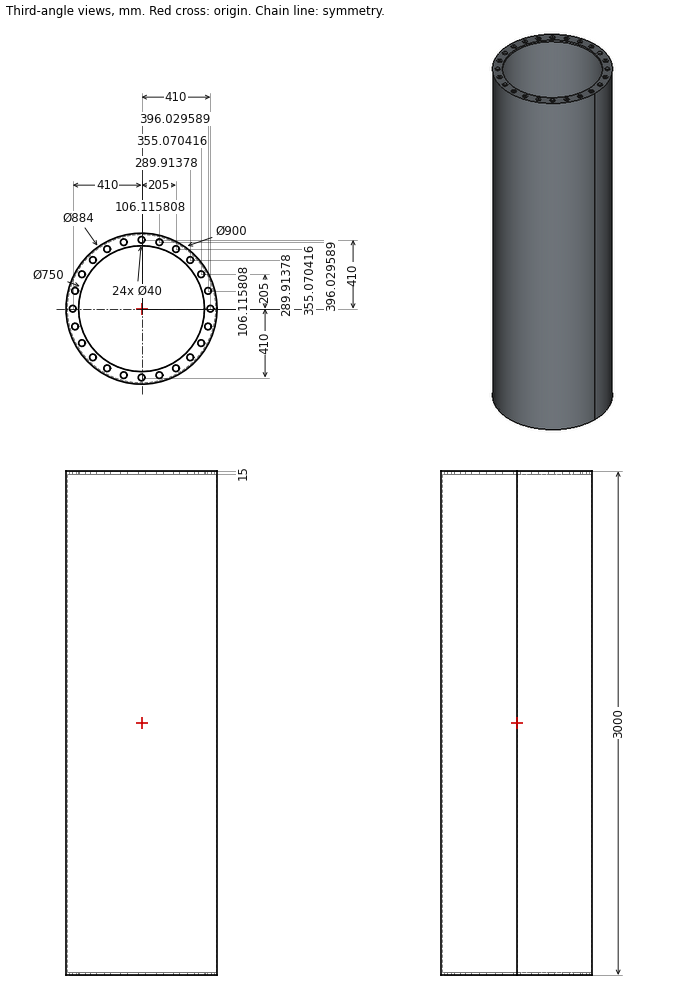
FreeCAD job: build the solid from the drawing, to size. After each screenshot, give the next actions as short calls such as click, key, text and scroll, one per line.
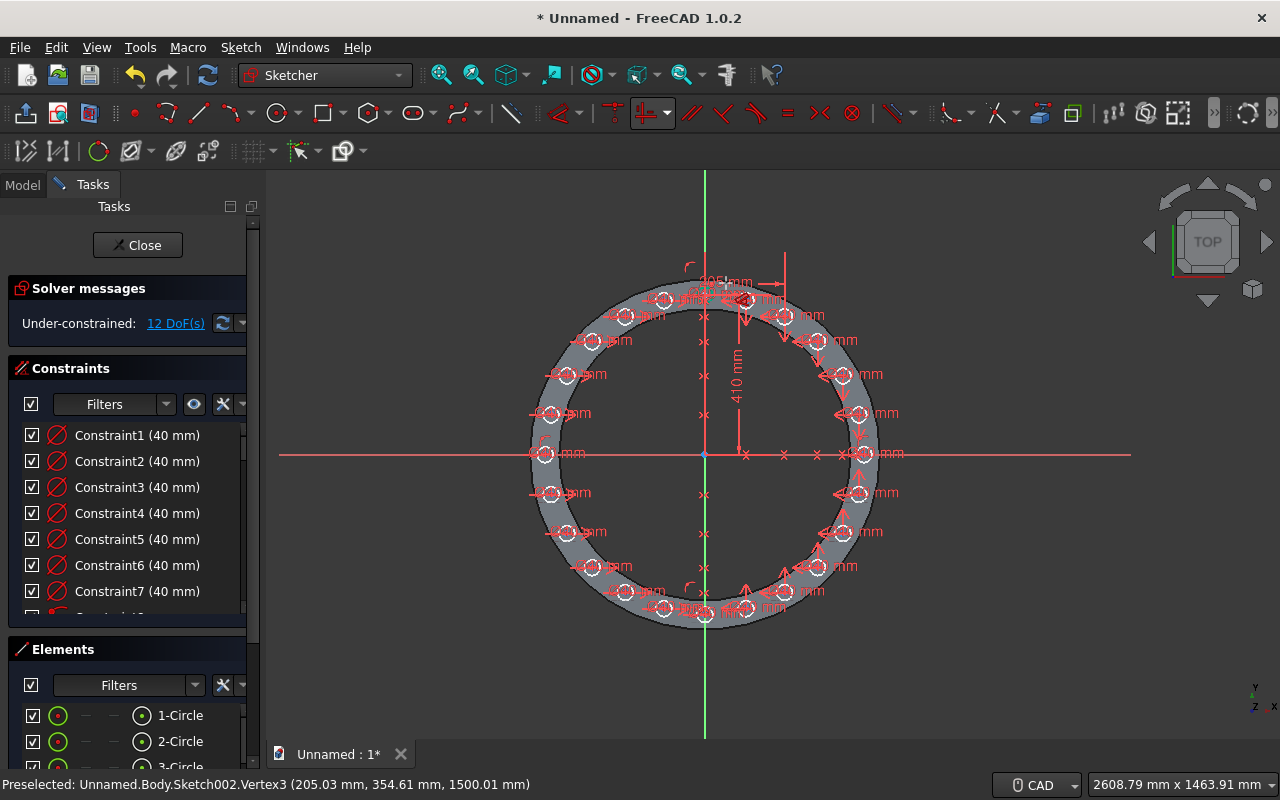
click(843, 376)
click(877, 397)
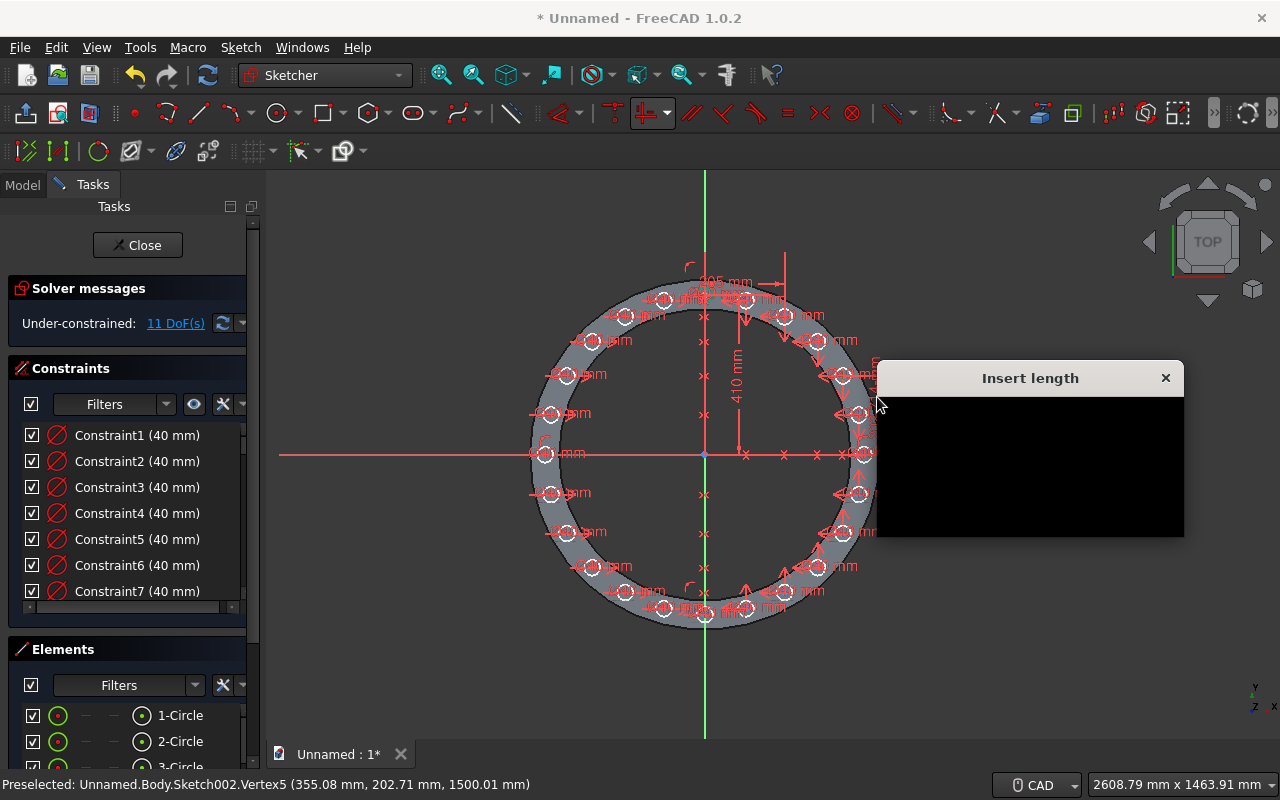
text(205)
key(Return)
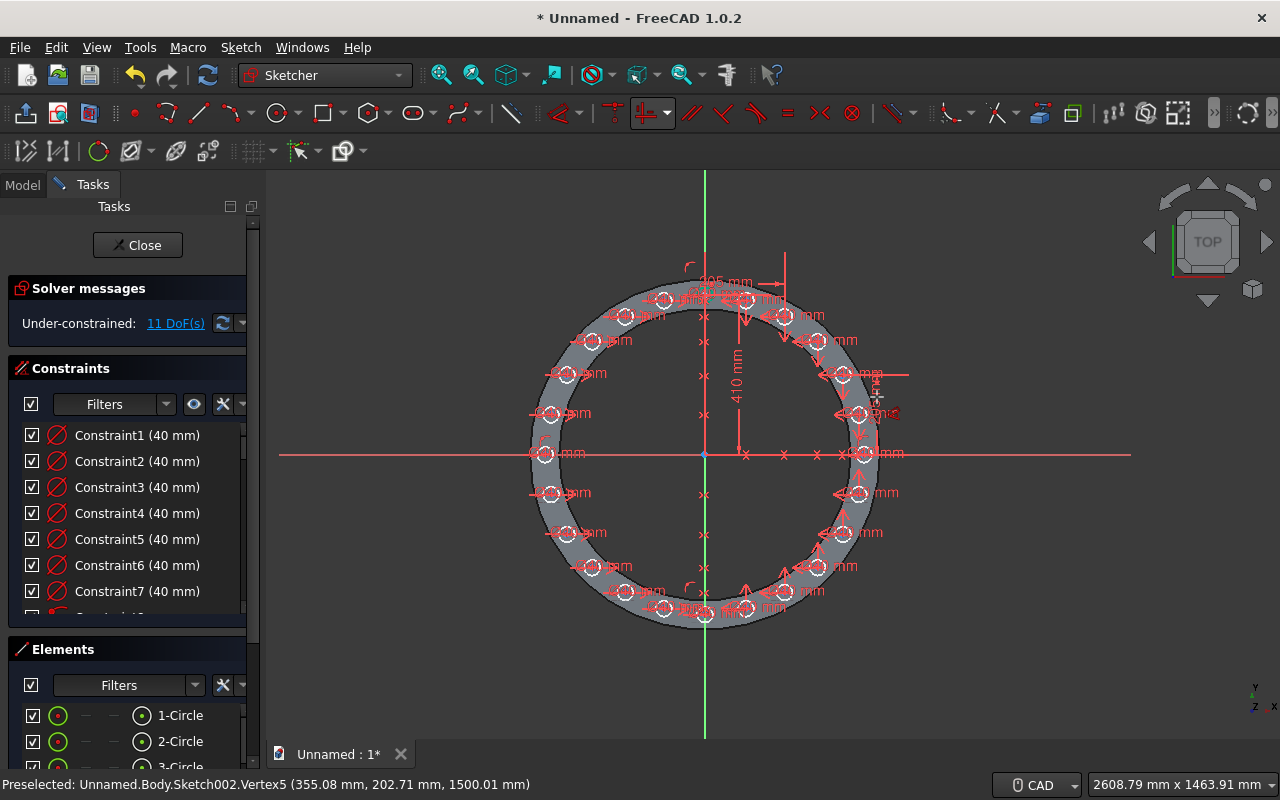
click(864, 455)
click(784, 489)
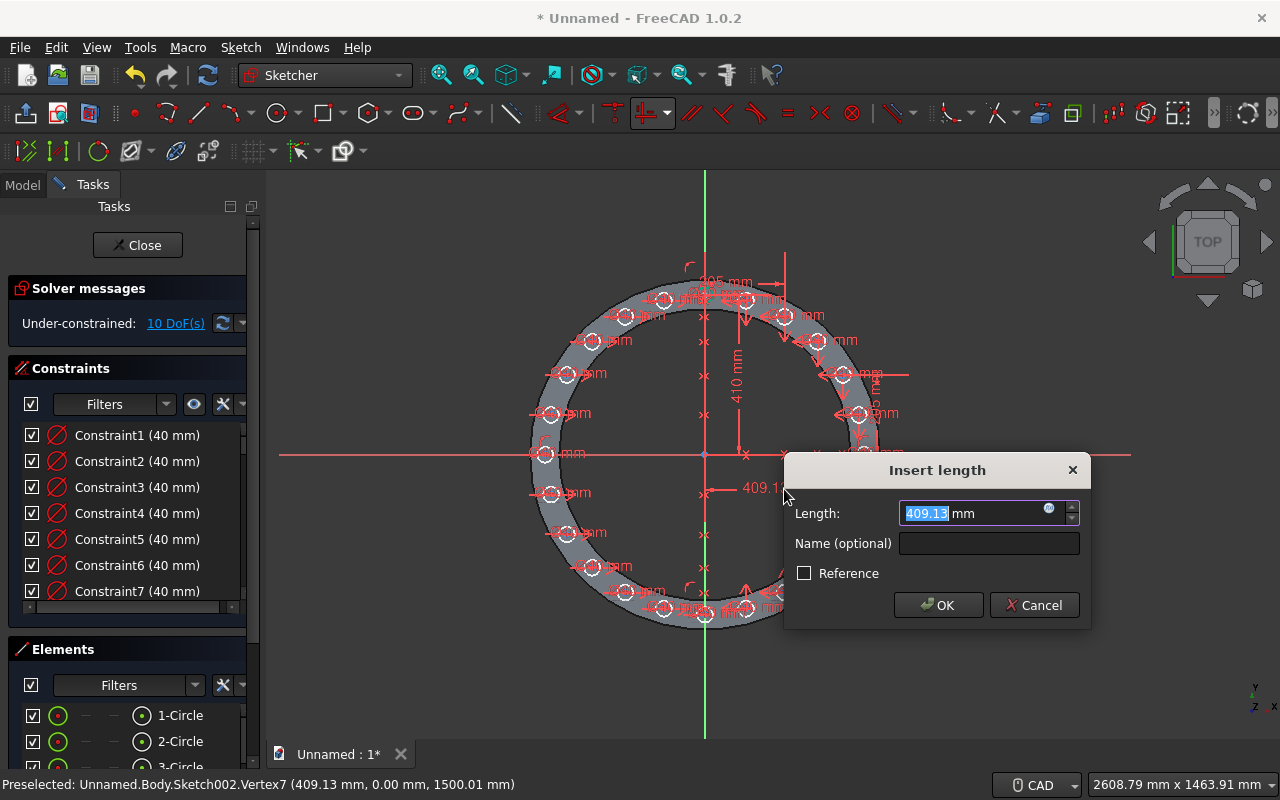
text(410)
key(Return)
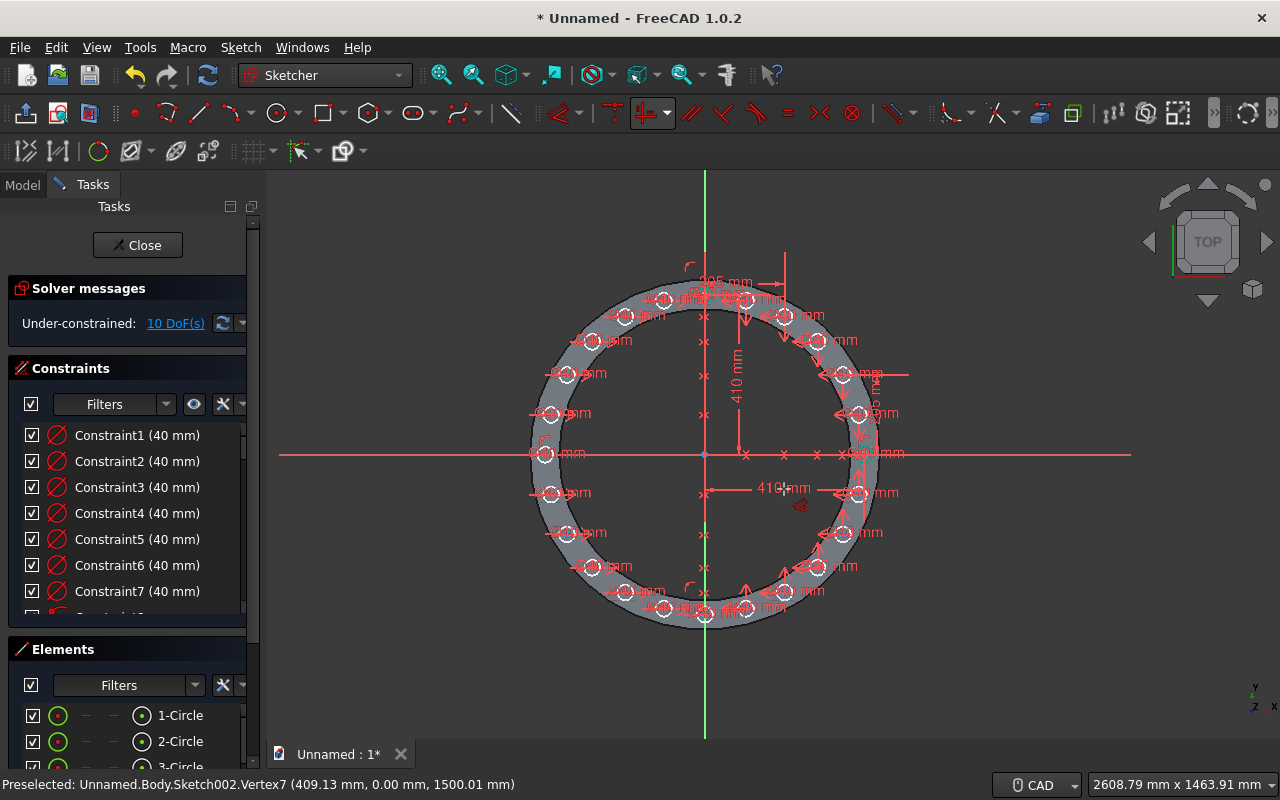
click(705, 615)
click(739, 535)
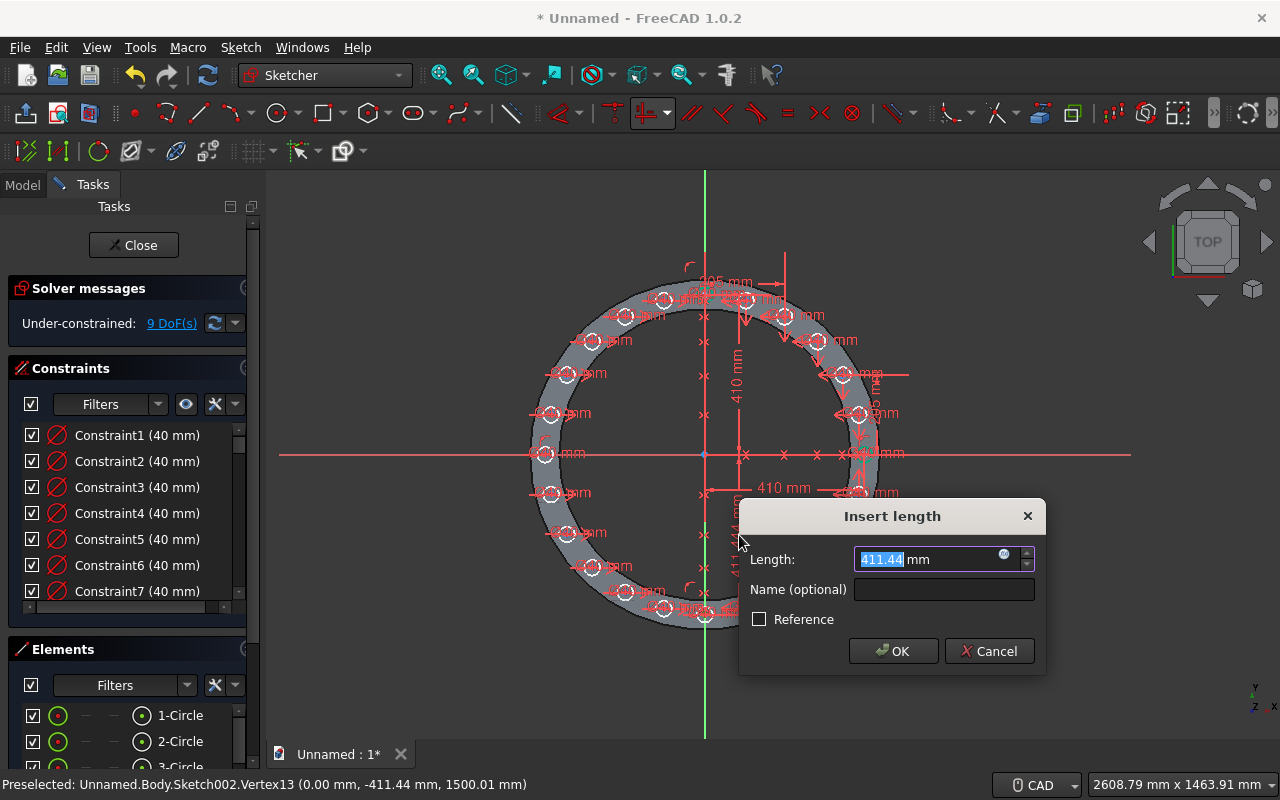
text(410)
key(Return)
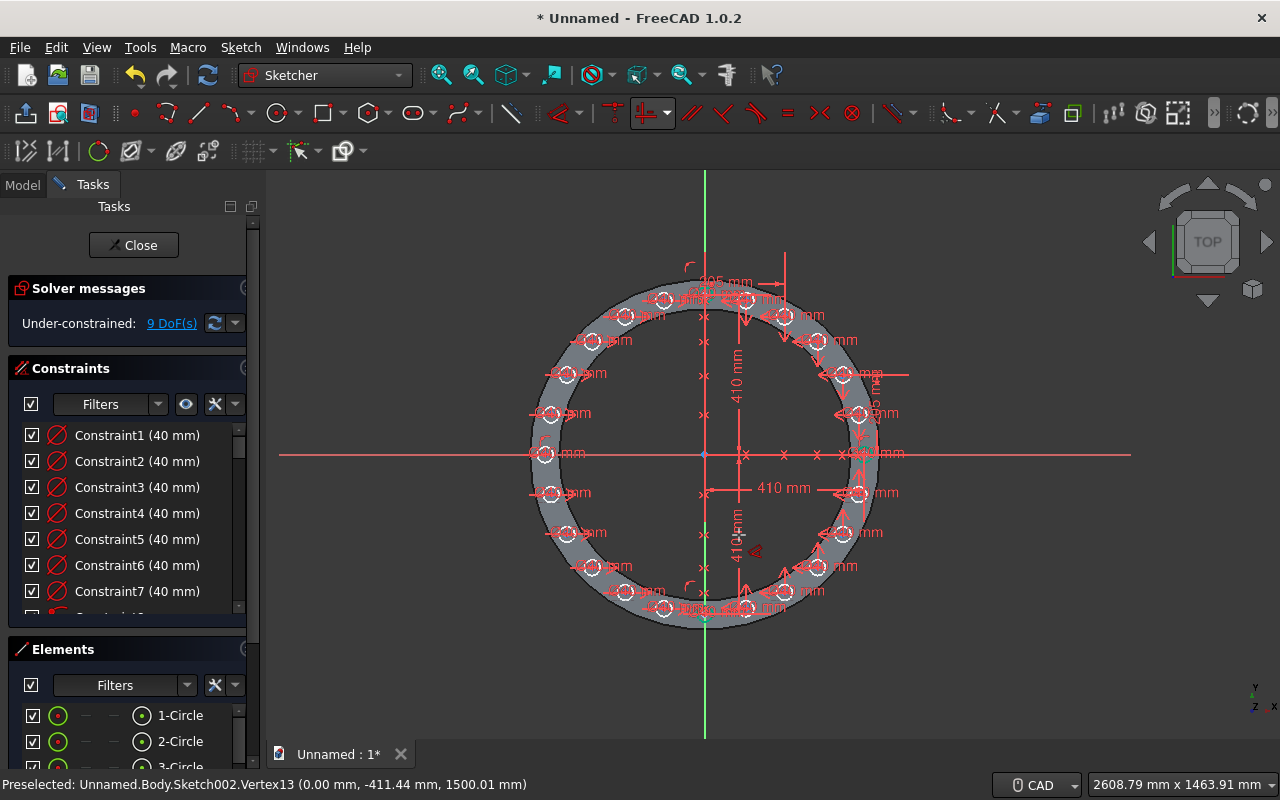
click(545, 455)
click(625, 489)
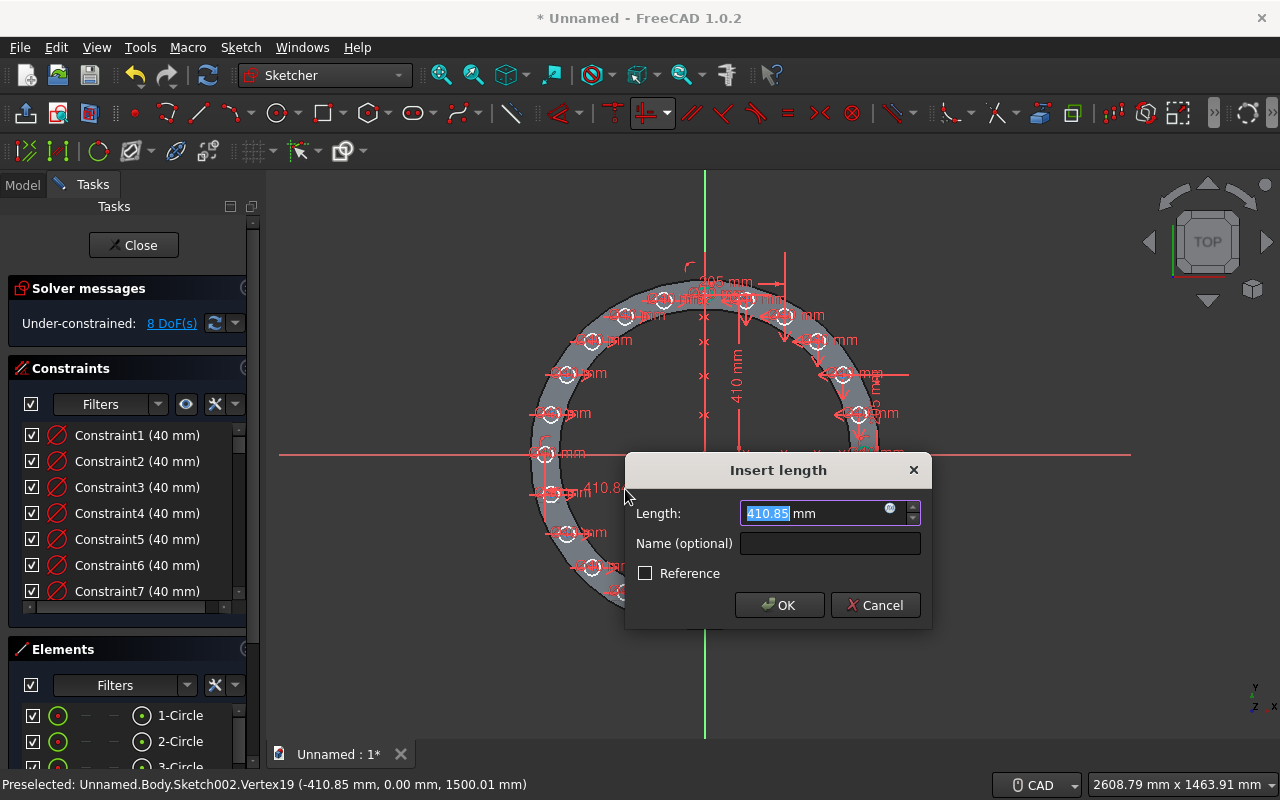
text(410)
key(Return)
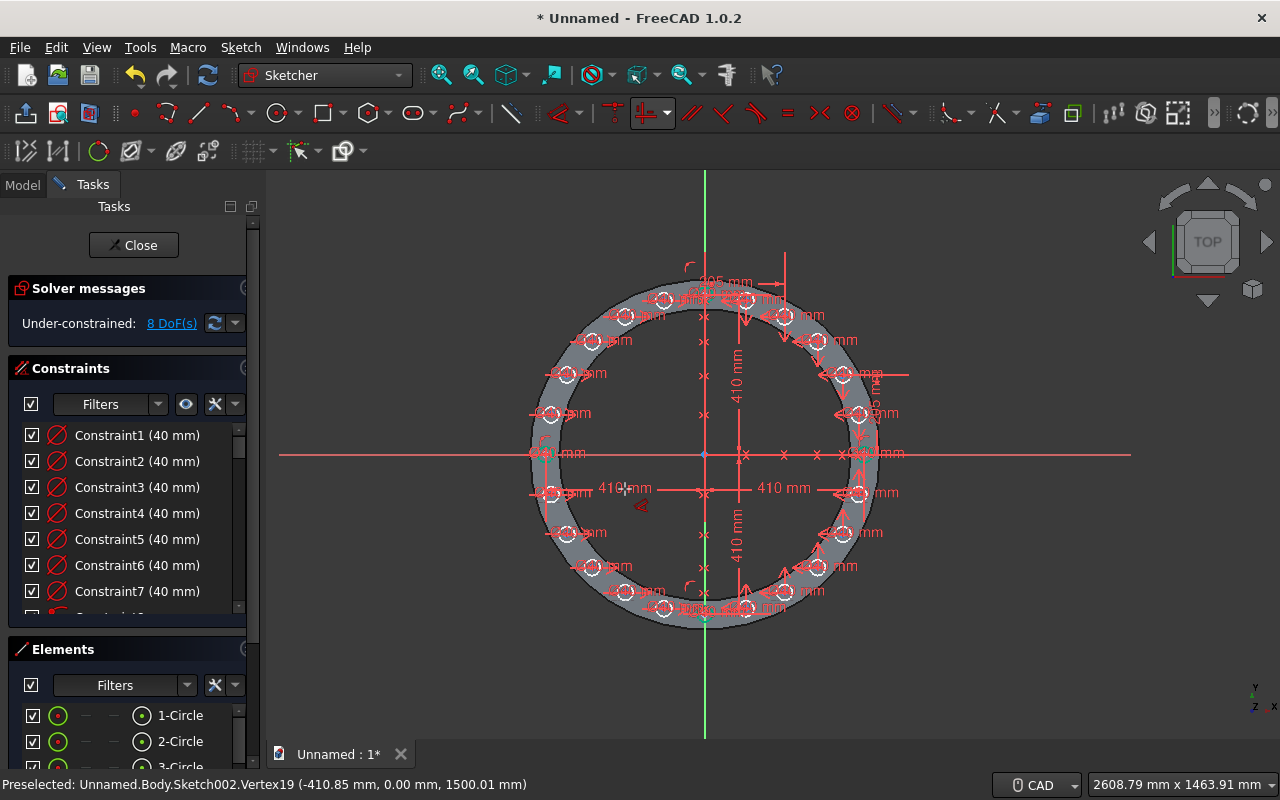
click(818, 342)
click(722, 308)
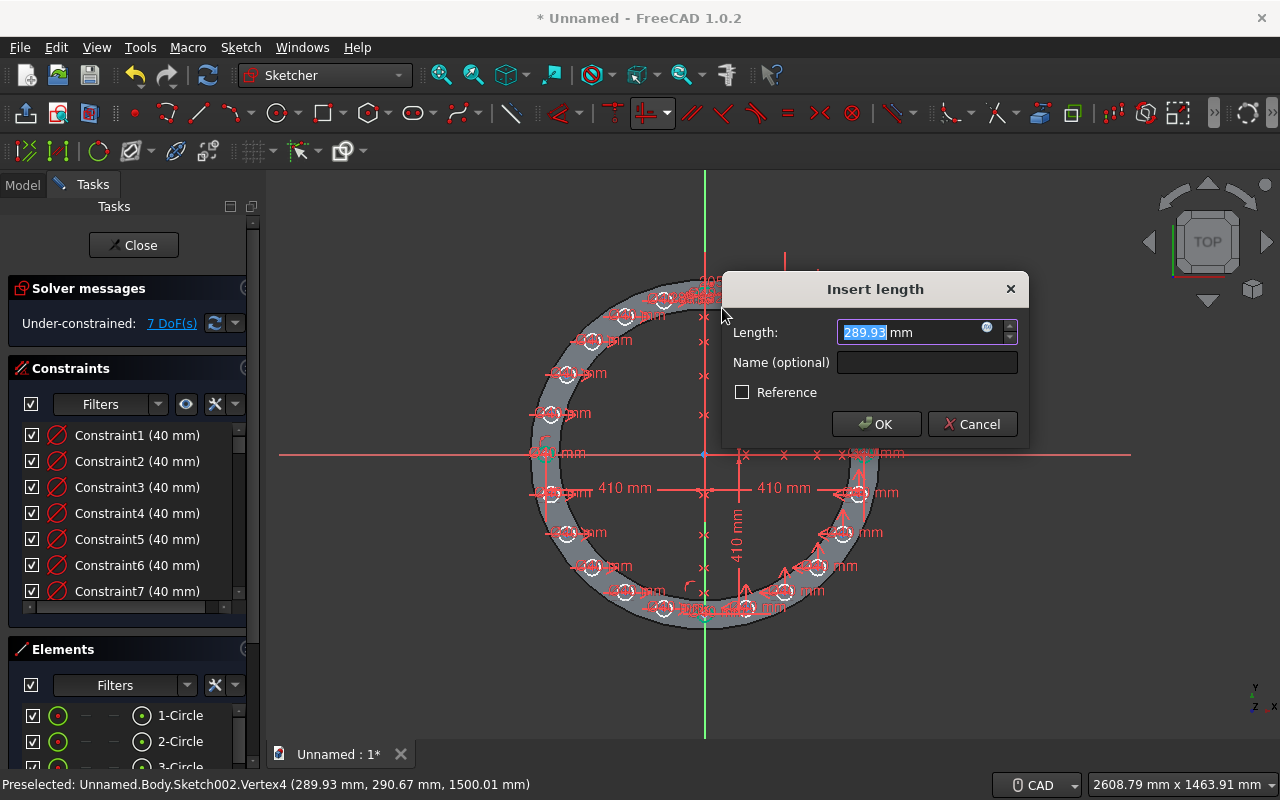
text(289.91378)
key(Return)